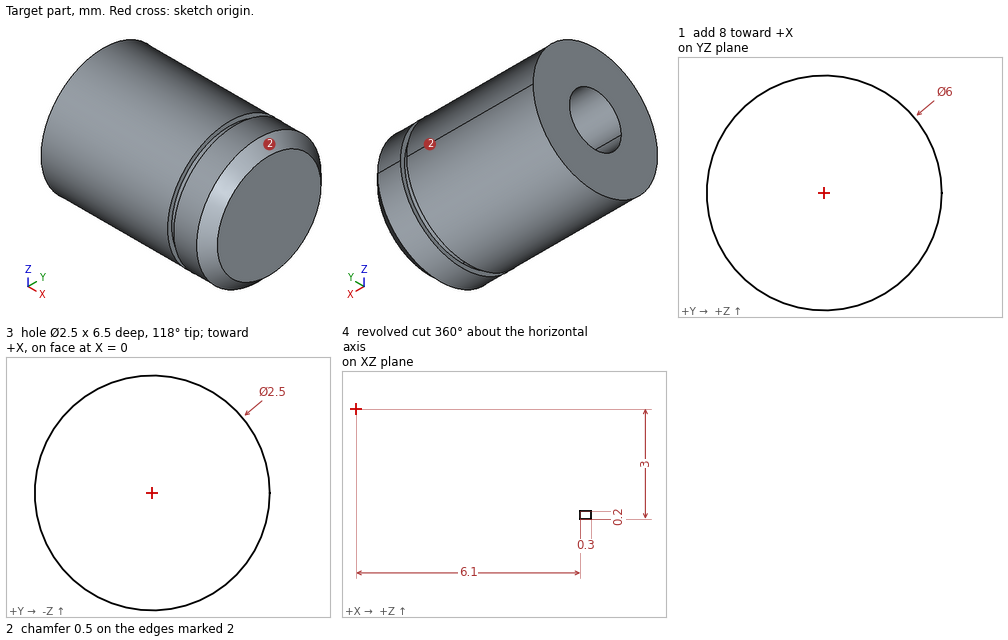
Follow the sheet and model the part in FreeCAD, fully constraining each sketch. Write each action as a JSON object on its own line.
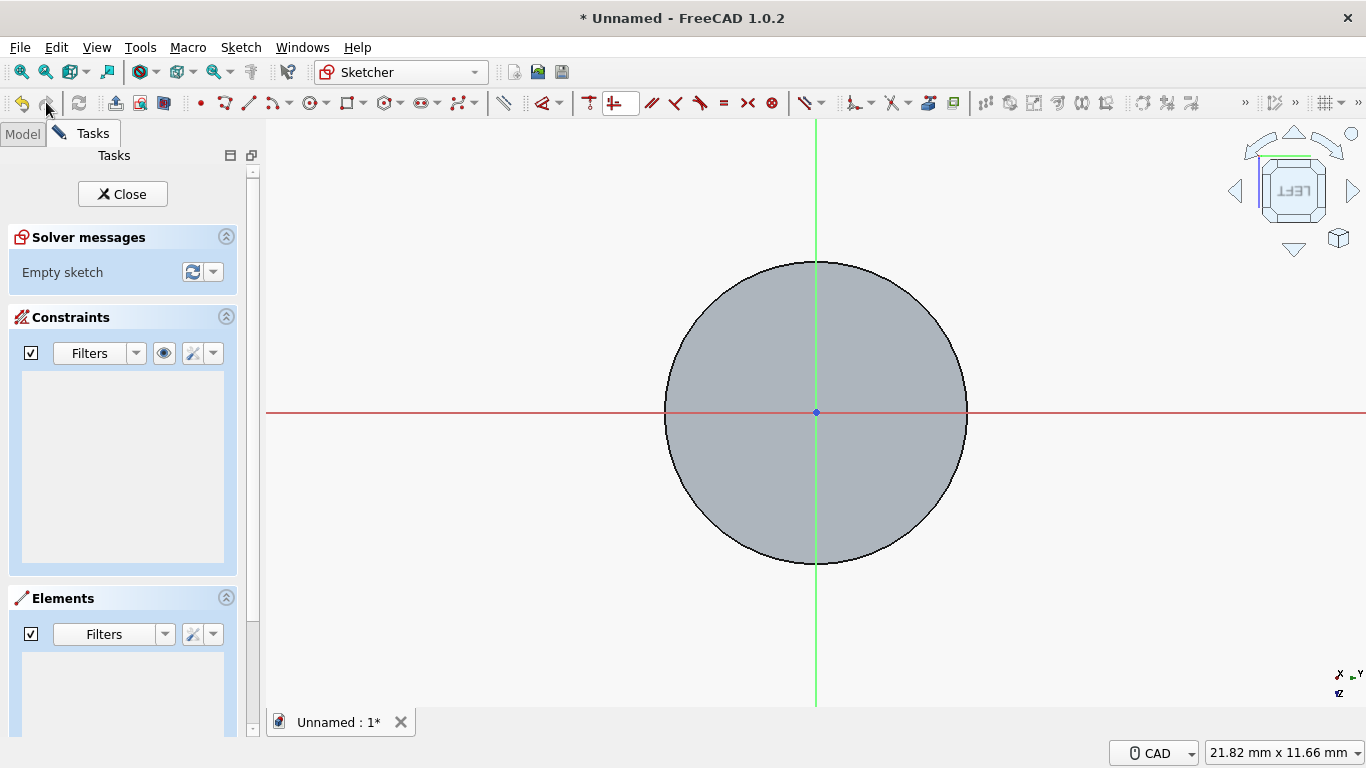
{"action": "scroll", "coordinate": [856, 413], "scroll_direction": "up", "scroll_amount": 5}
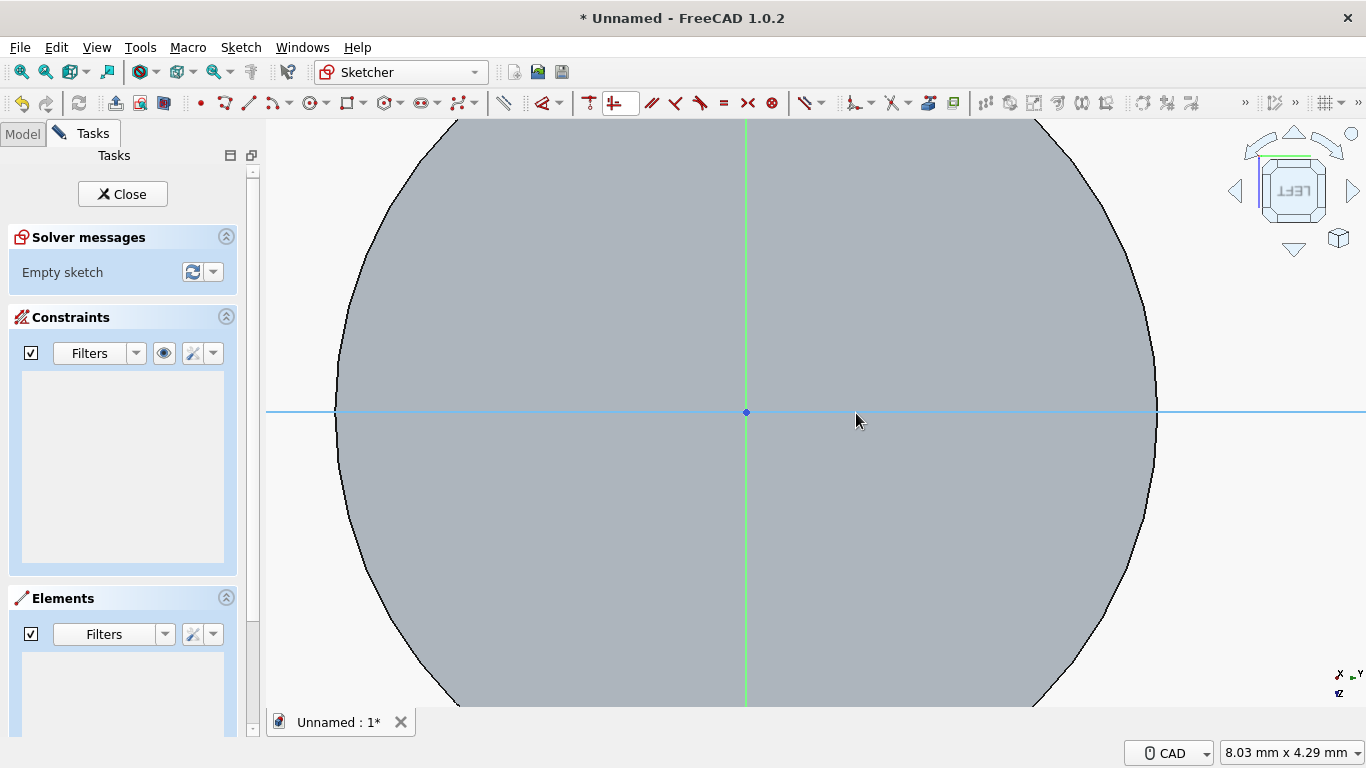
{"action": "key", "text": "g c"}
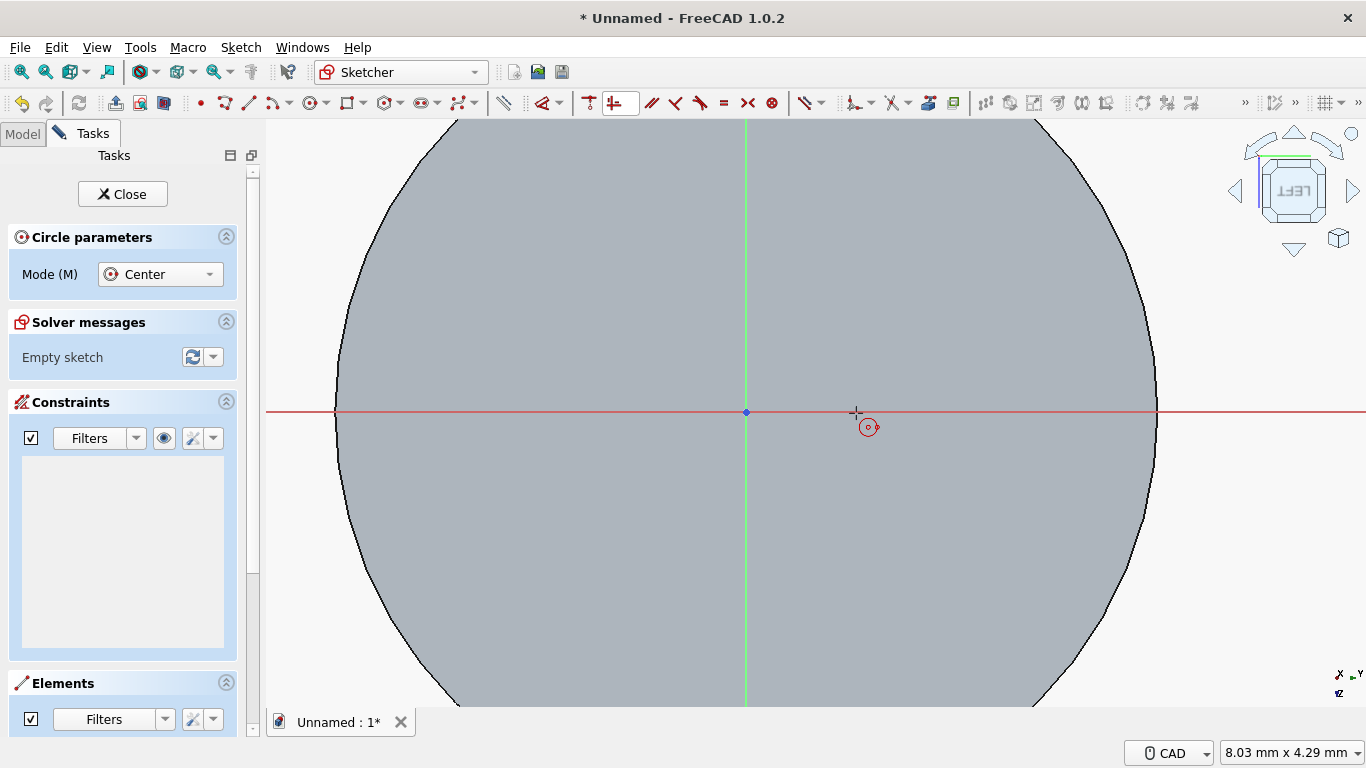
{"action": "left_click", "coordinate": [746, 412]}
{"action": "mouse_move", "coordinate": [867, 291]}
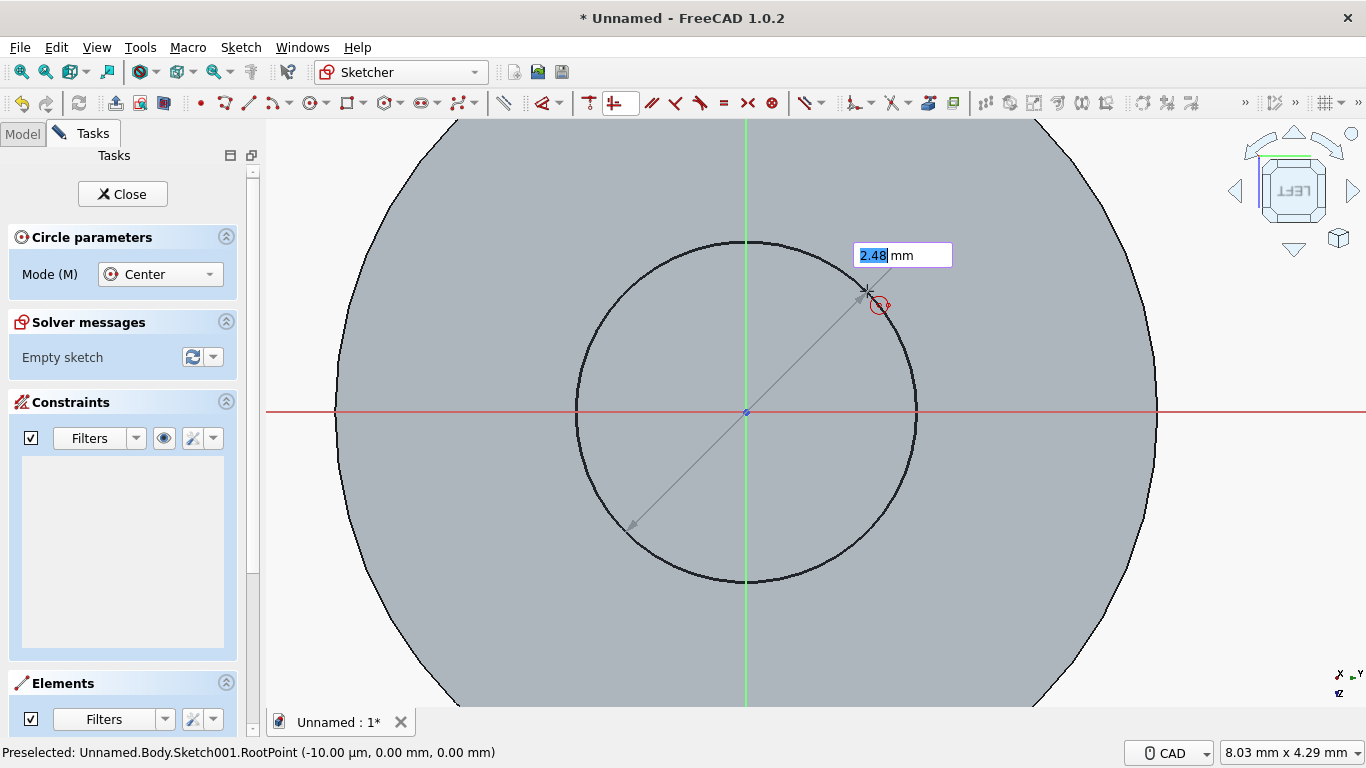
{"action": "type", "text": "2.5"}
{"action": "key", "text": "Return"}
{"action": "key", "text": "Escape"}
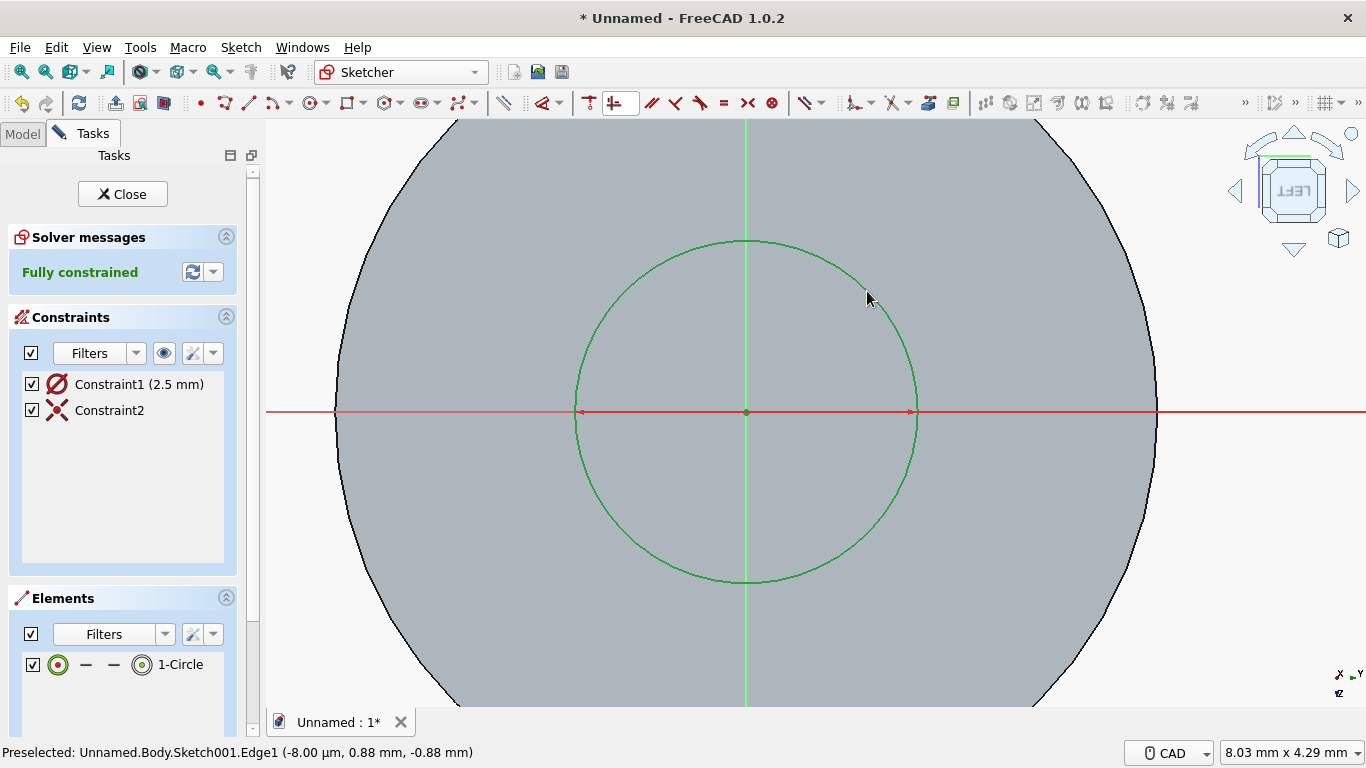
{"action": "left_click", "coordinate": [123, 194]}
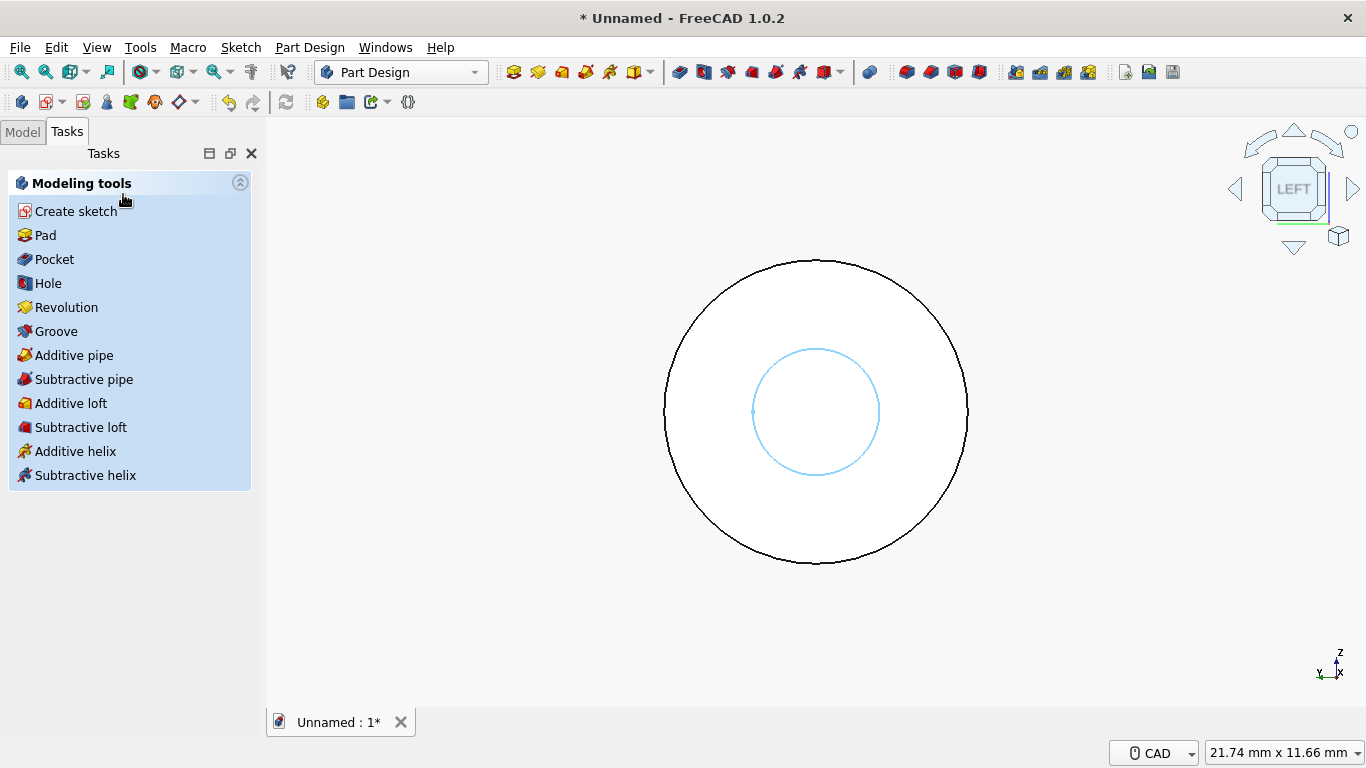
{"action": "left_click", "coordinate": [704, 72]}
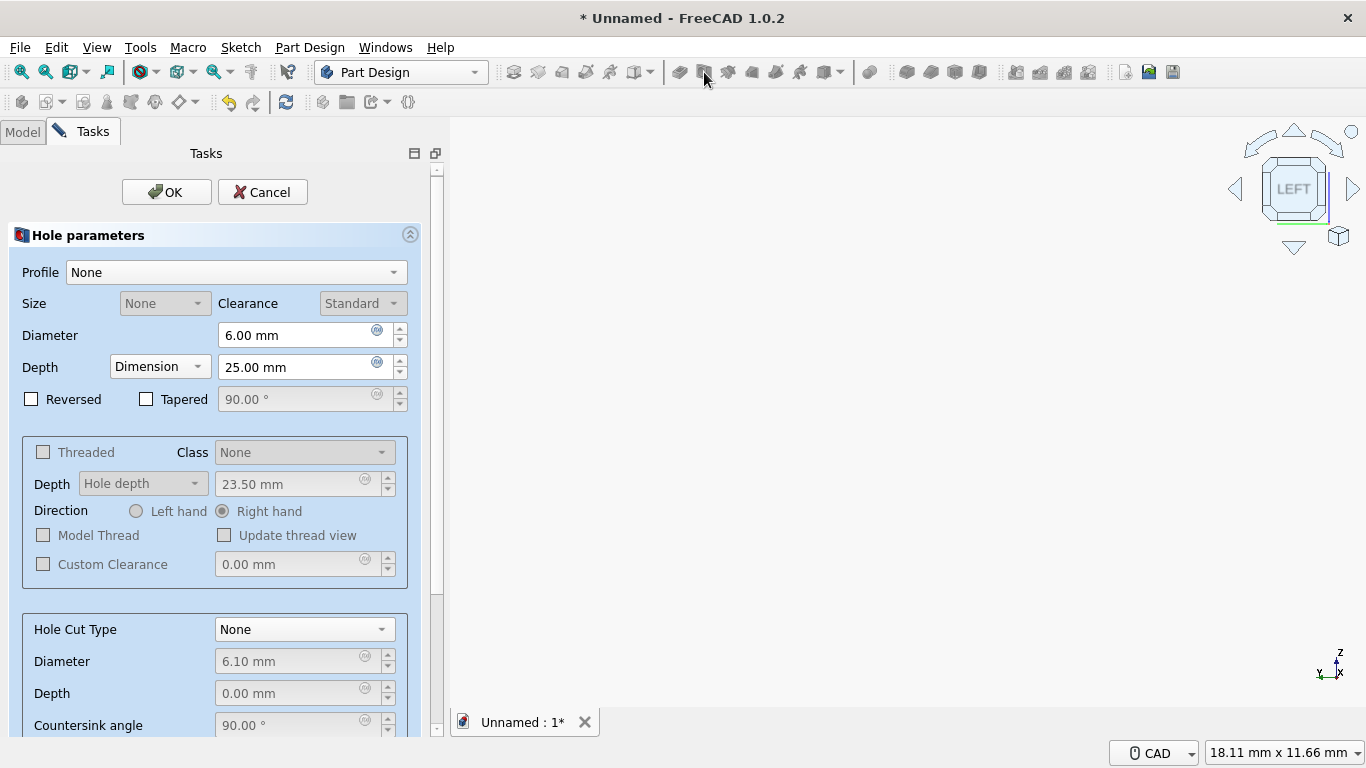
{"action": "triple_click", "coordinate": [305, 335]}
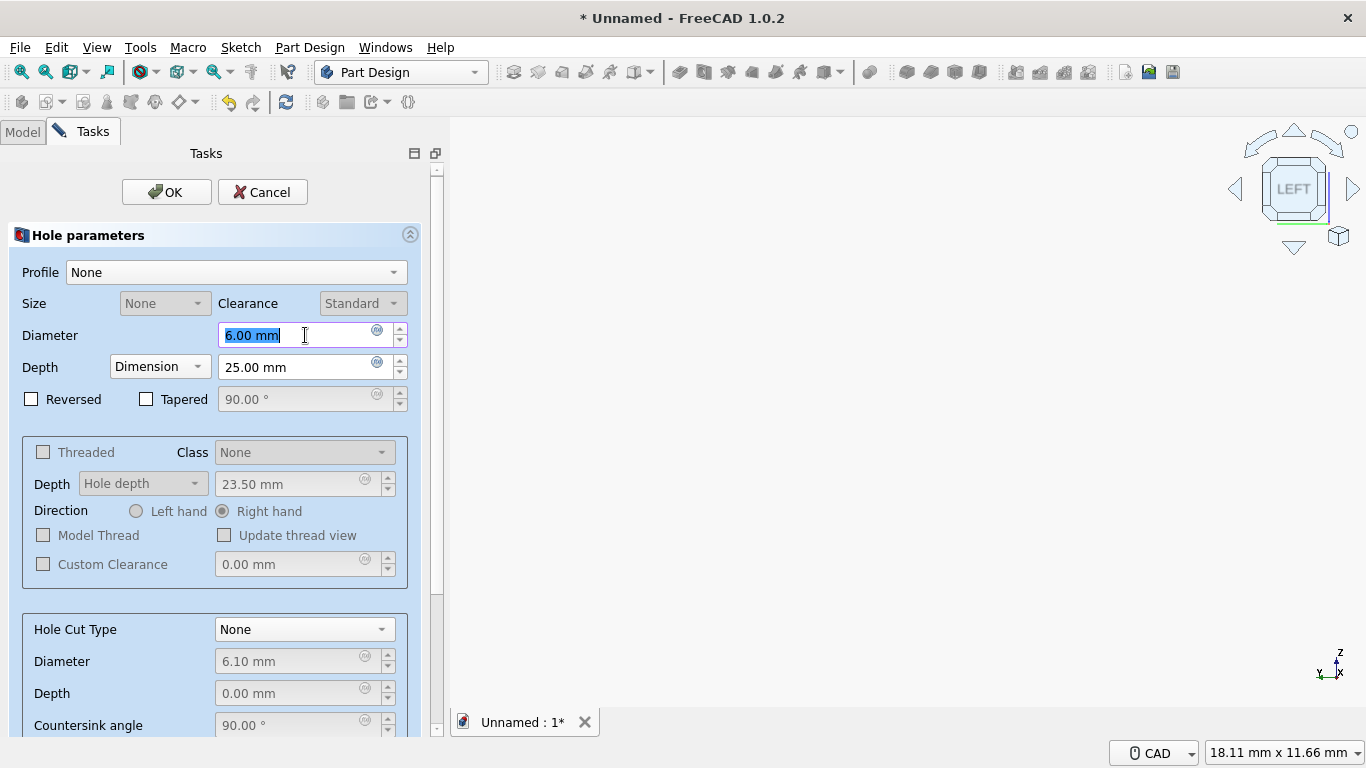
{"action": "type", "text": "2.5"}
{"action": "key", "text": "Tab"}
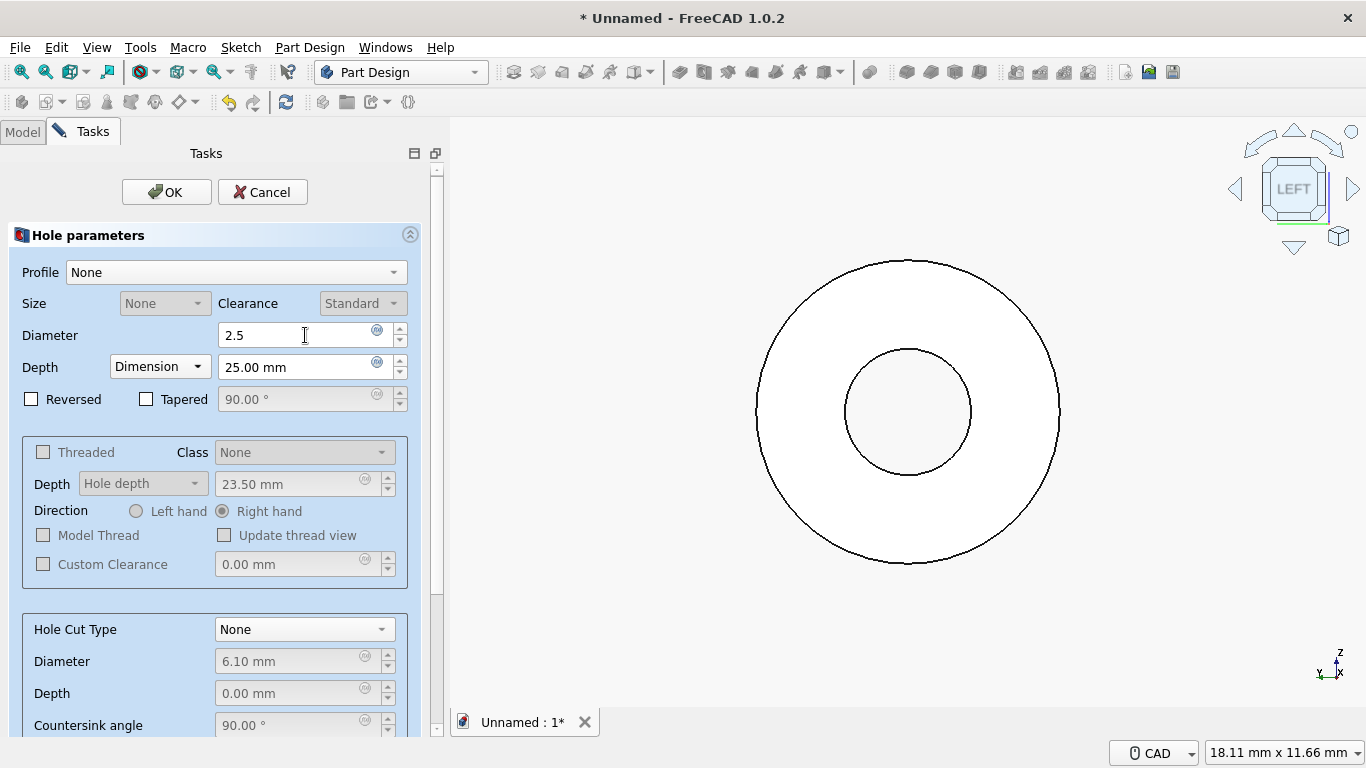
{"action": "triple_click", "coordinate": [305, 367]}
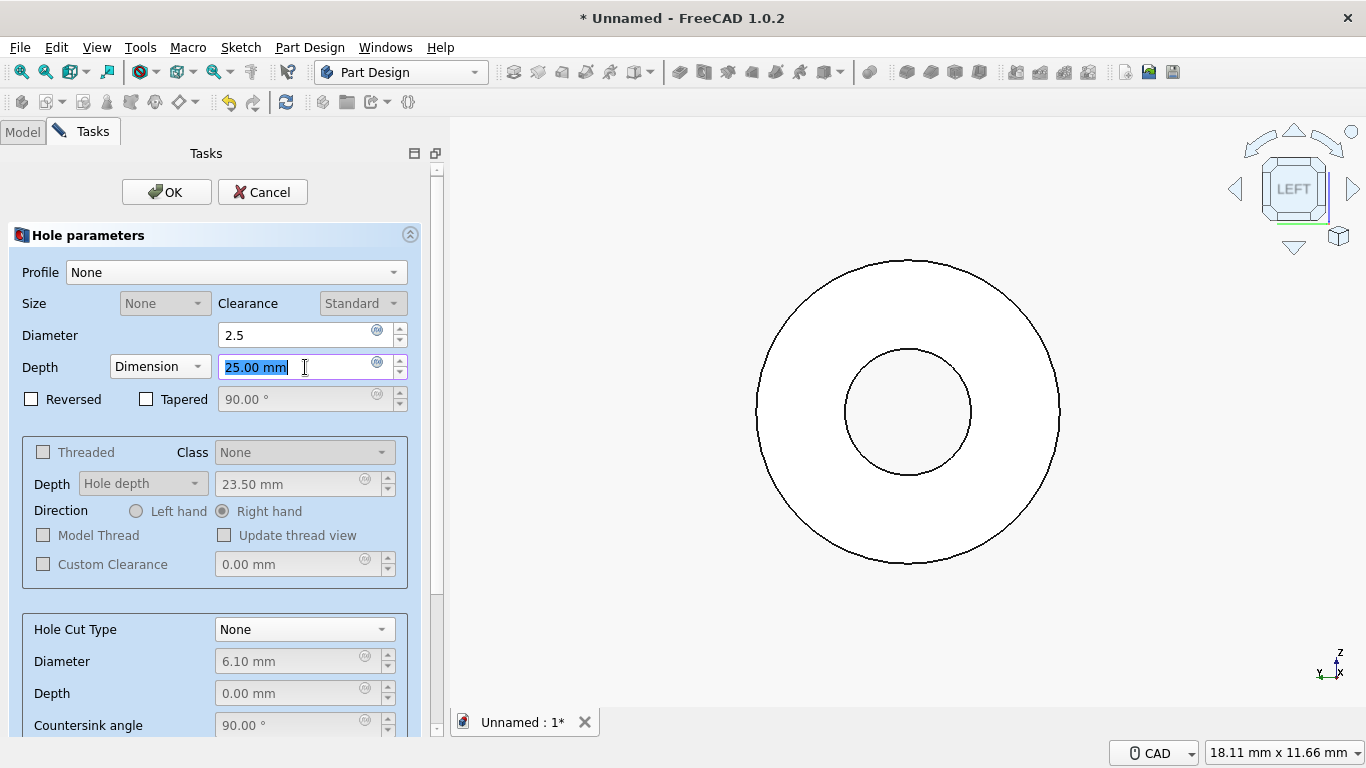
{"action": "type", "text": "6.5"}
{"action": "key", "text": "Tab"}